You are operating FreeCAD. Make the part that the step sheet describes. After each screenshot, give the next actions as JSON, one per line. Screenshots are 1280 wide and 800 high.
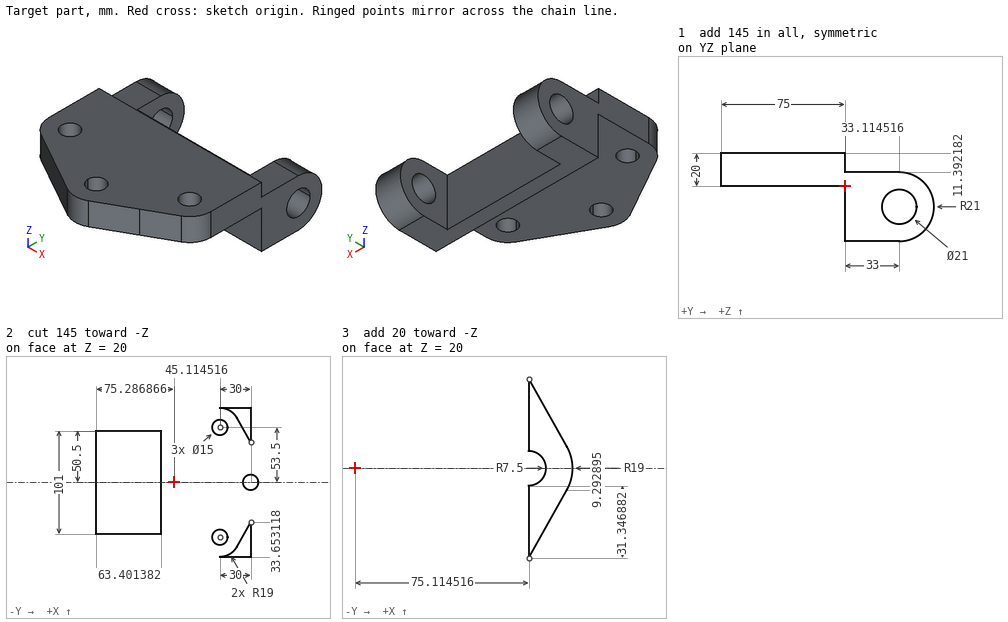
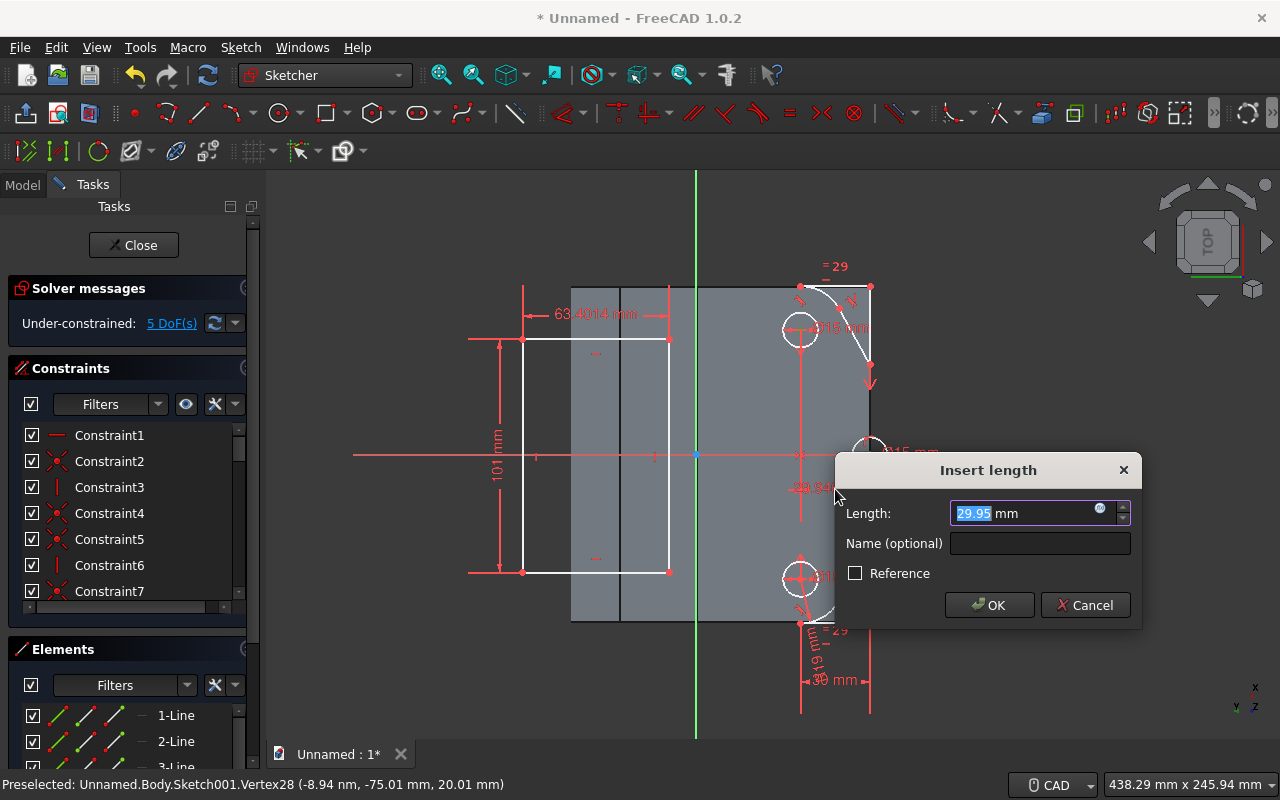
{"action": "type", "text": "30"}
{"action": "key", "text": "Return"}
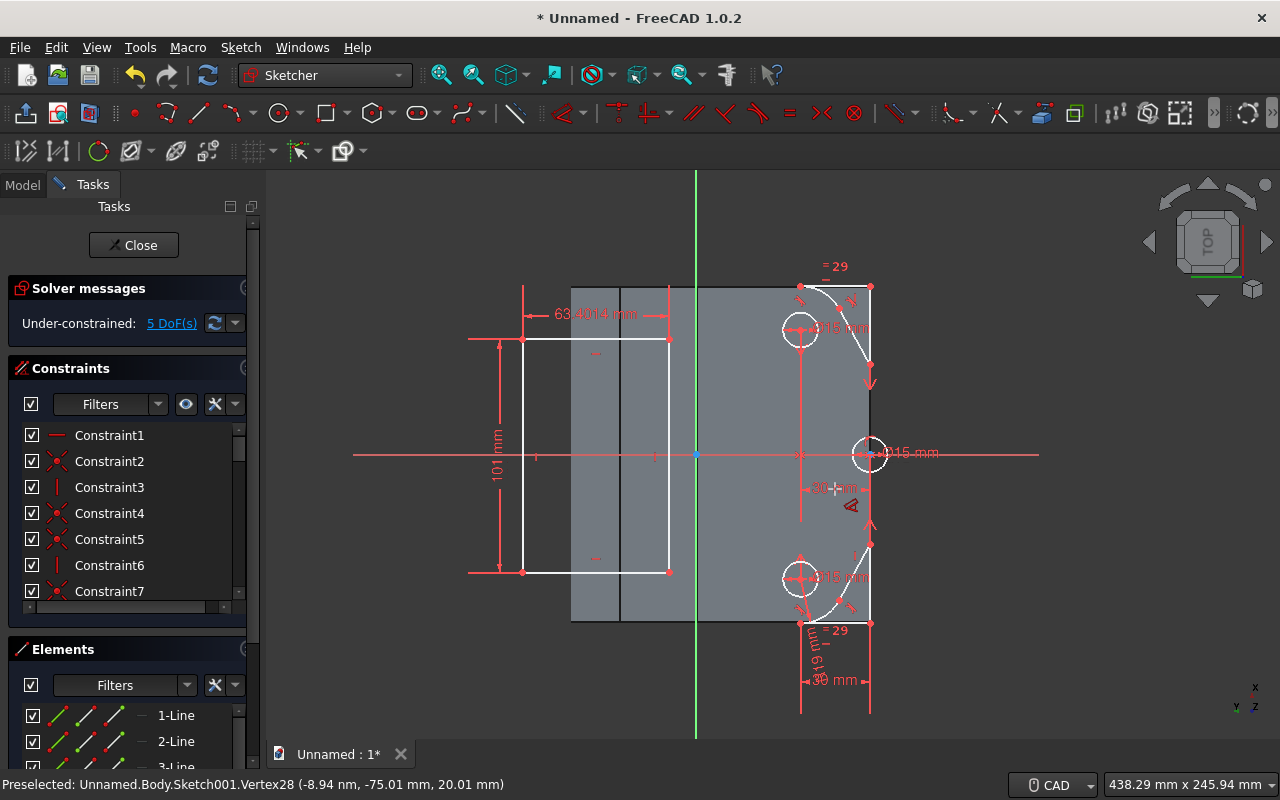
{"action": "left_click", "coordinate": [801, 330]}
{"action": "left_click", "coordinate": [835, 392]}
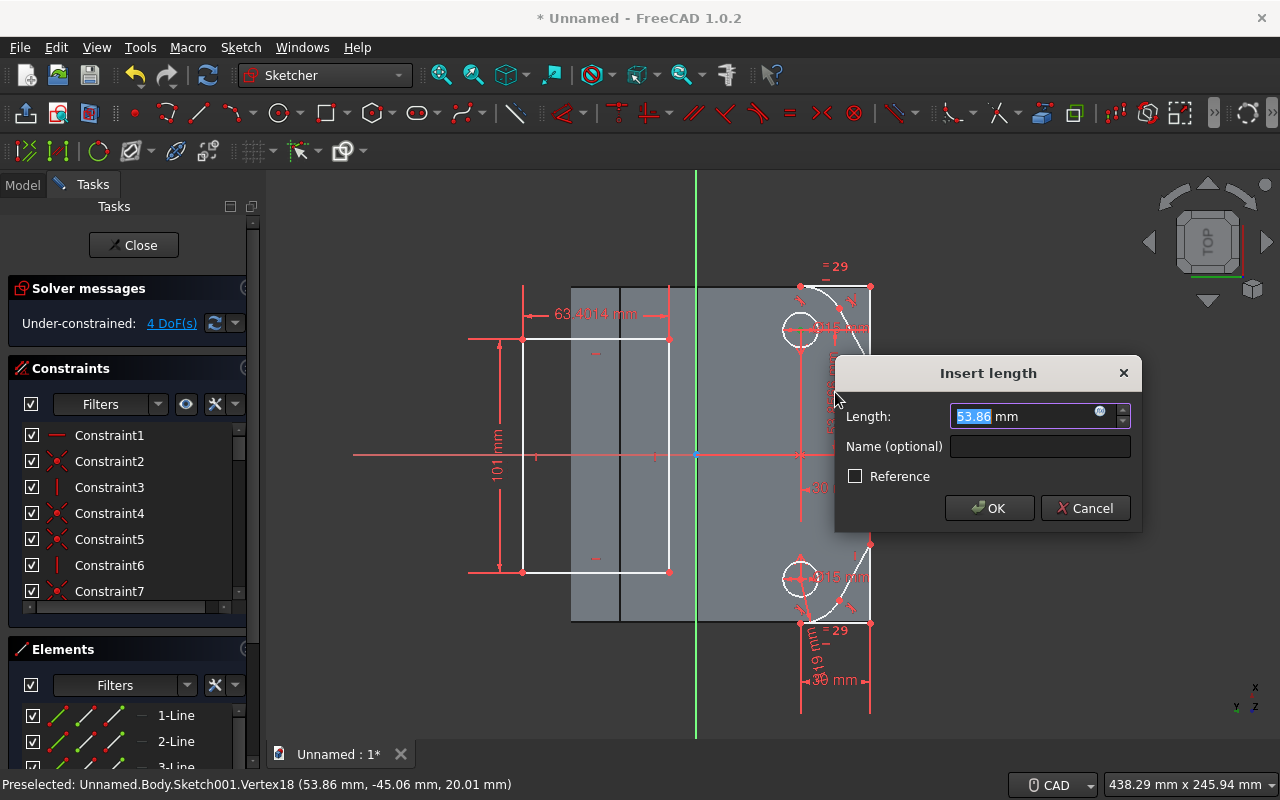
{"action": "type", "text": "53.5"}
{"action": "key", "text": "Return"}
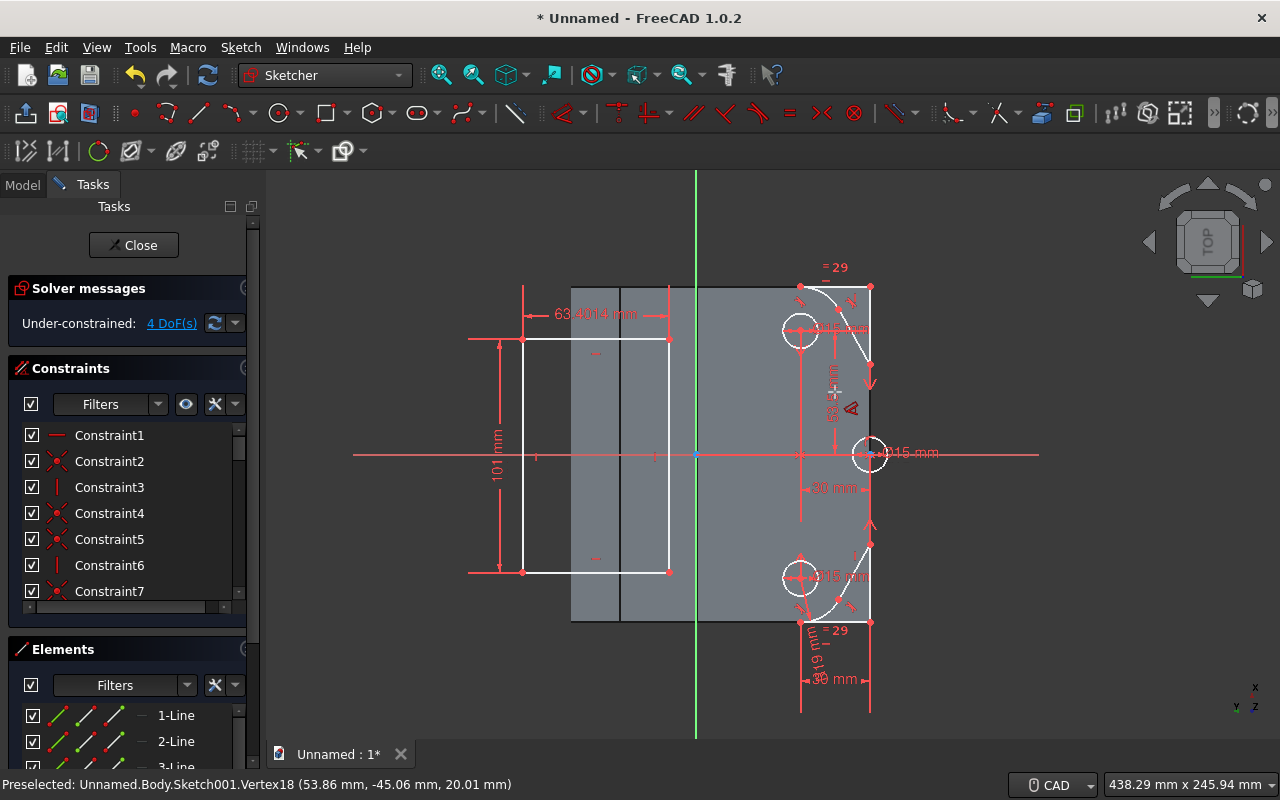
{"action": "left_click", "coordinate": [523, 339]}
{"action": "left_click", "coordinate": [489, 397]}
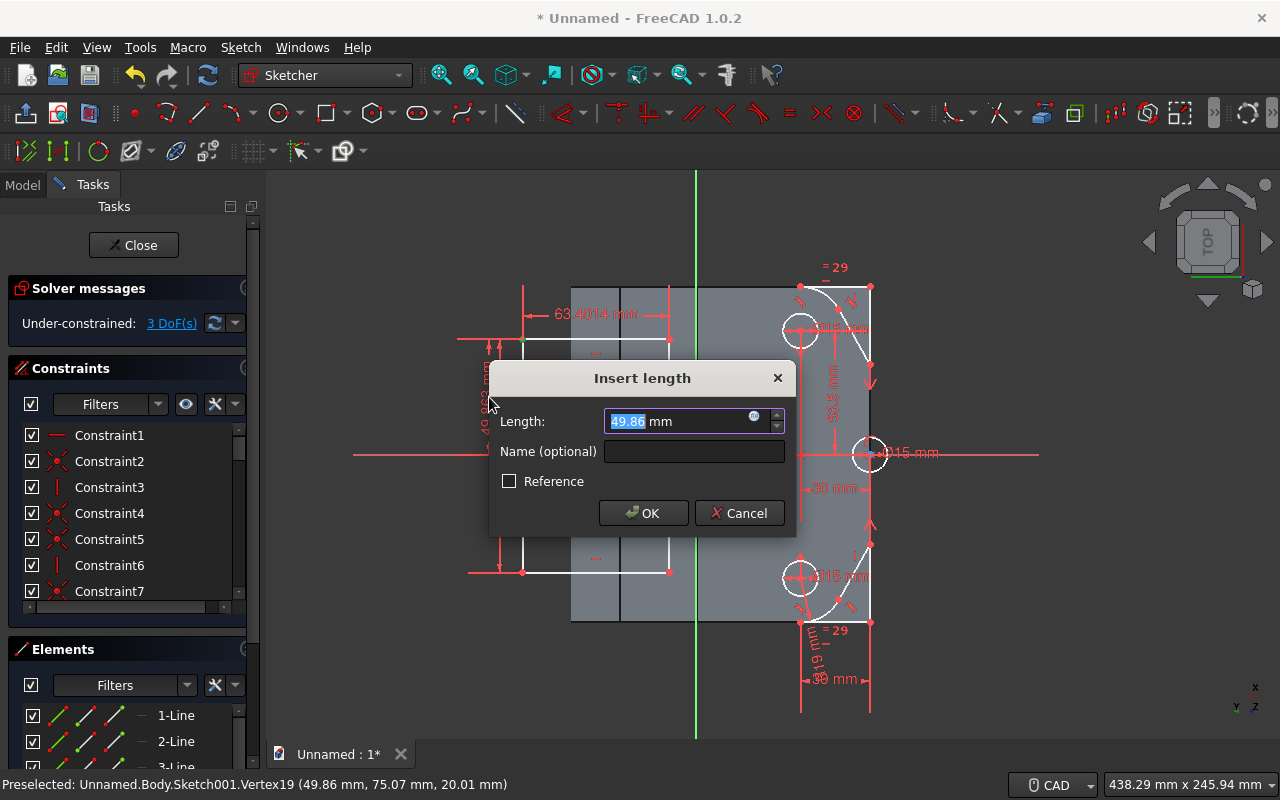
{"action": "type", "text": "50.5"}
{"action": "key", "text": "Return"}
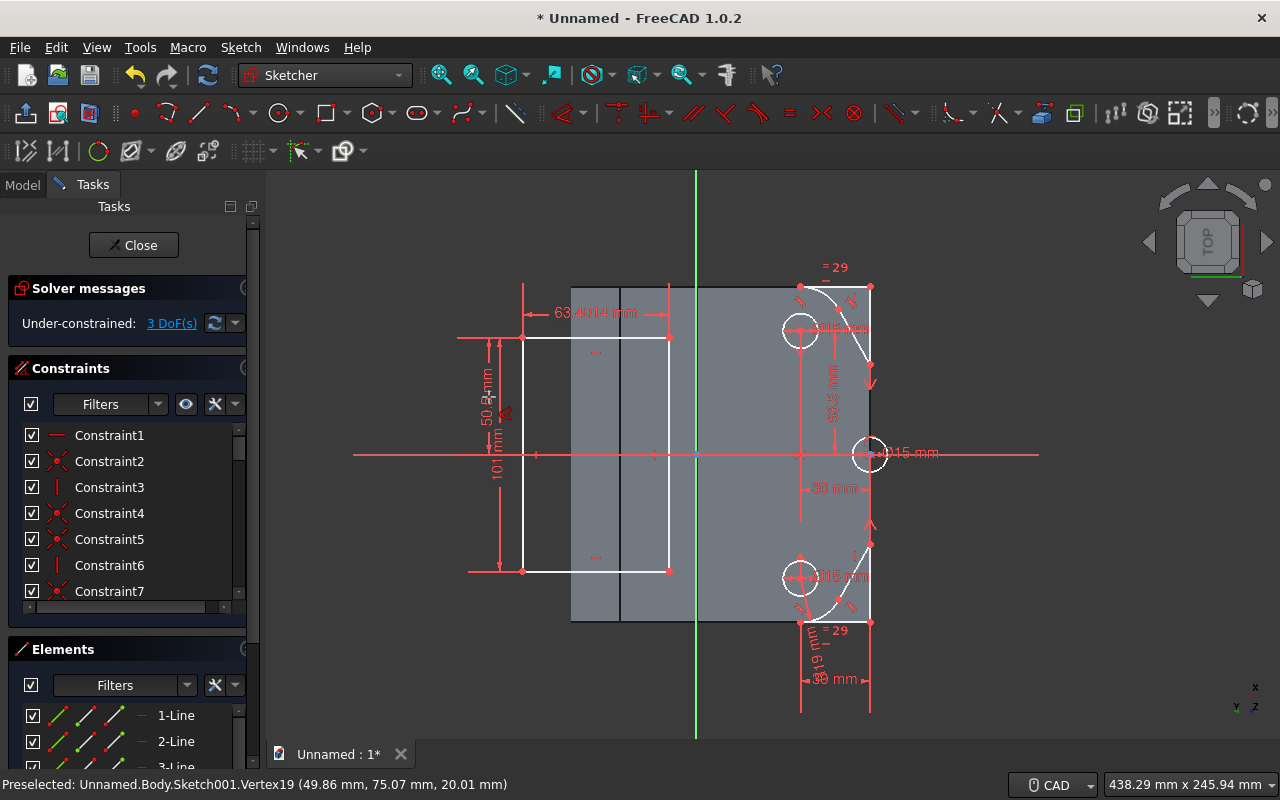
{"action": "left_click", "coordinate": [870, 599]}
{"action": "left_click", "coordinate": [904, 583]}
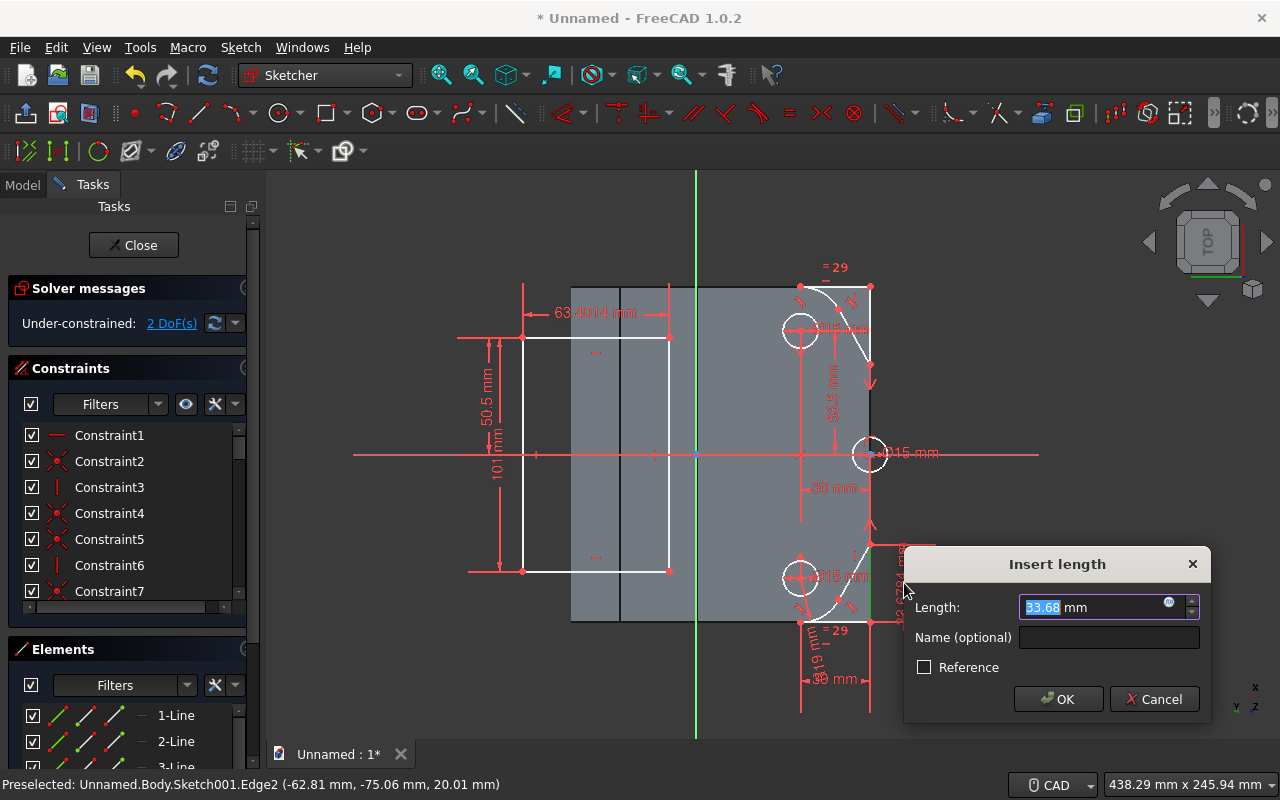
{"action": "type", "text": "33.653118"}
{"action": "key", "text": "Return"}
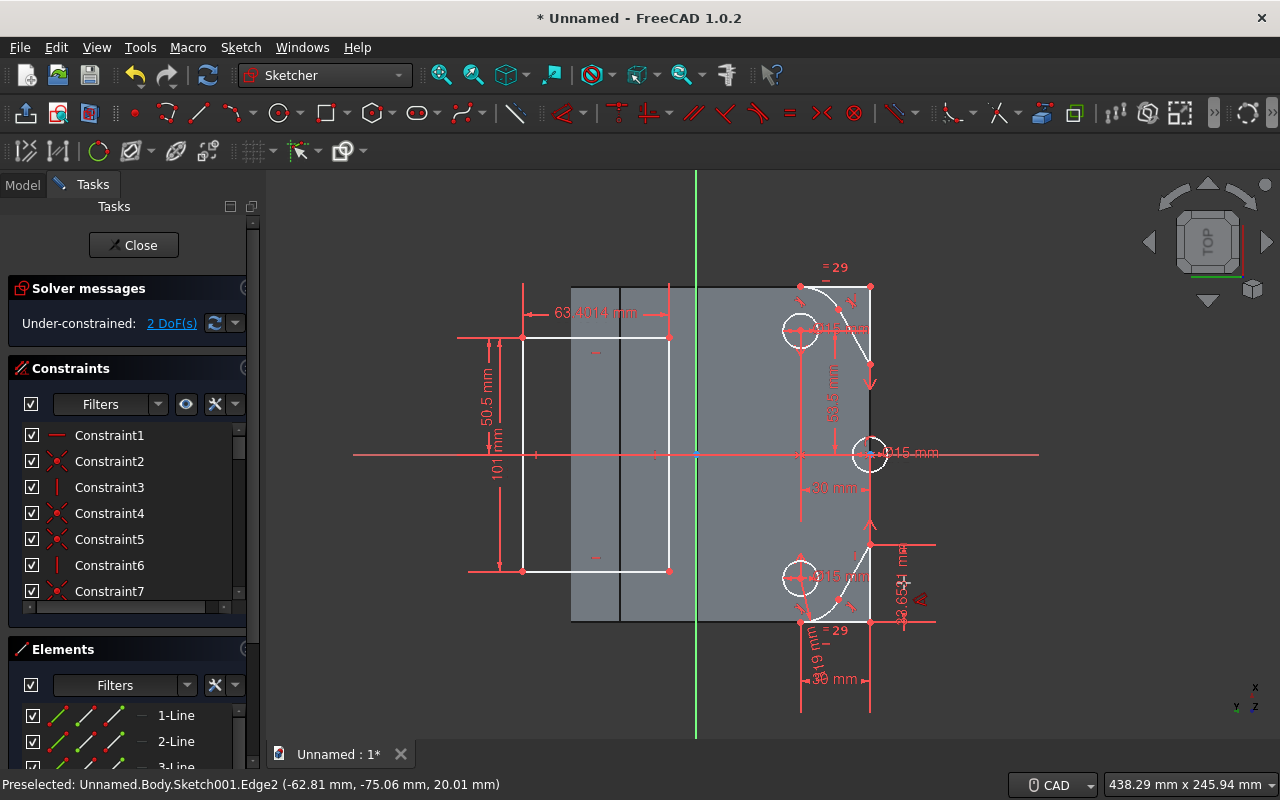
{"action": "left_click", "coordinate": [801, 331]}
{"action": "left_click", "coordinate": [748, 297]}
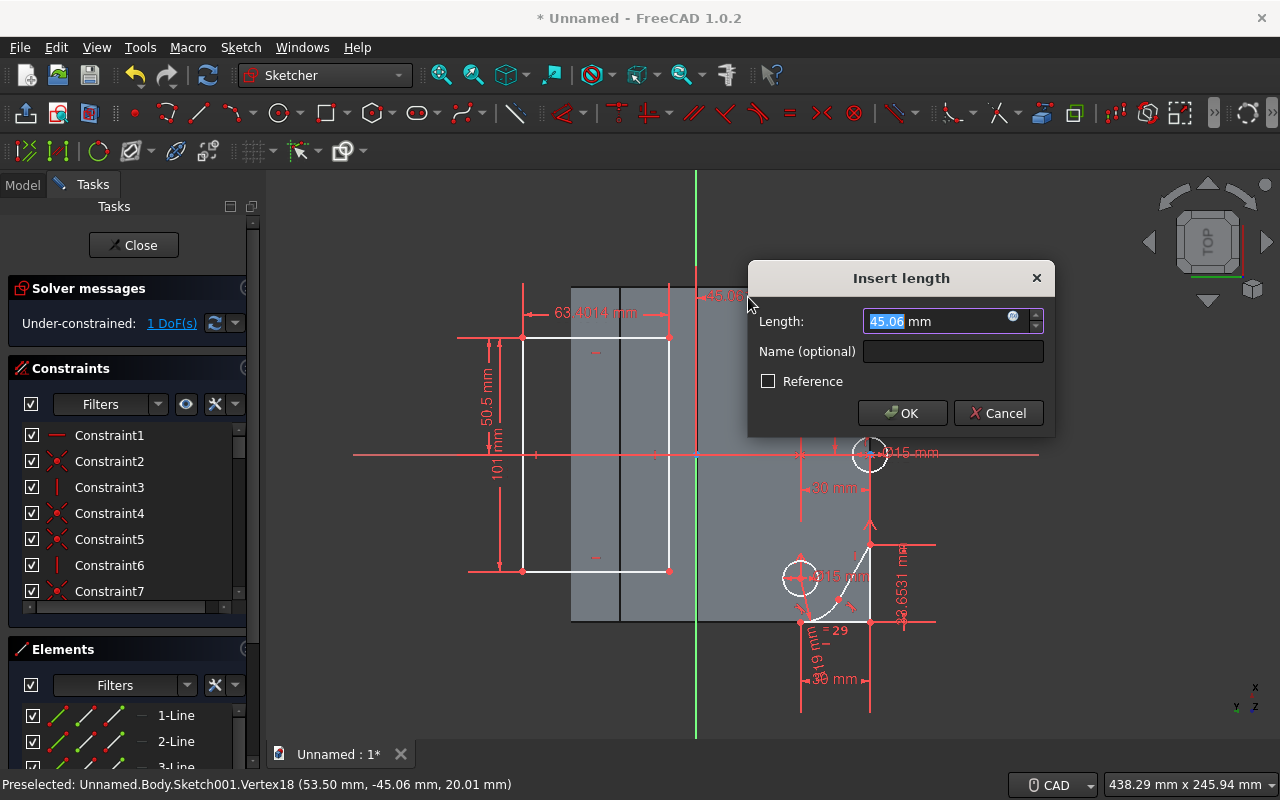
{"action": "type", "text": "45.114516"}
{"action": "key", "text": "Return"}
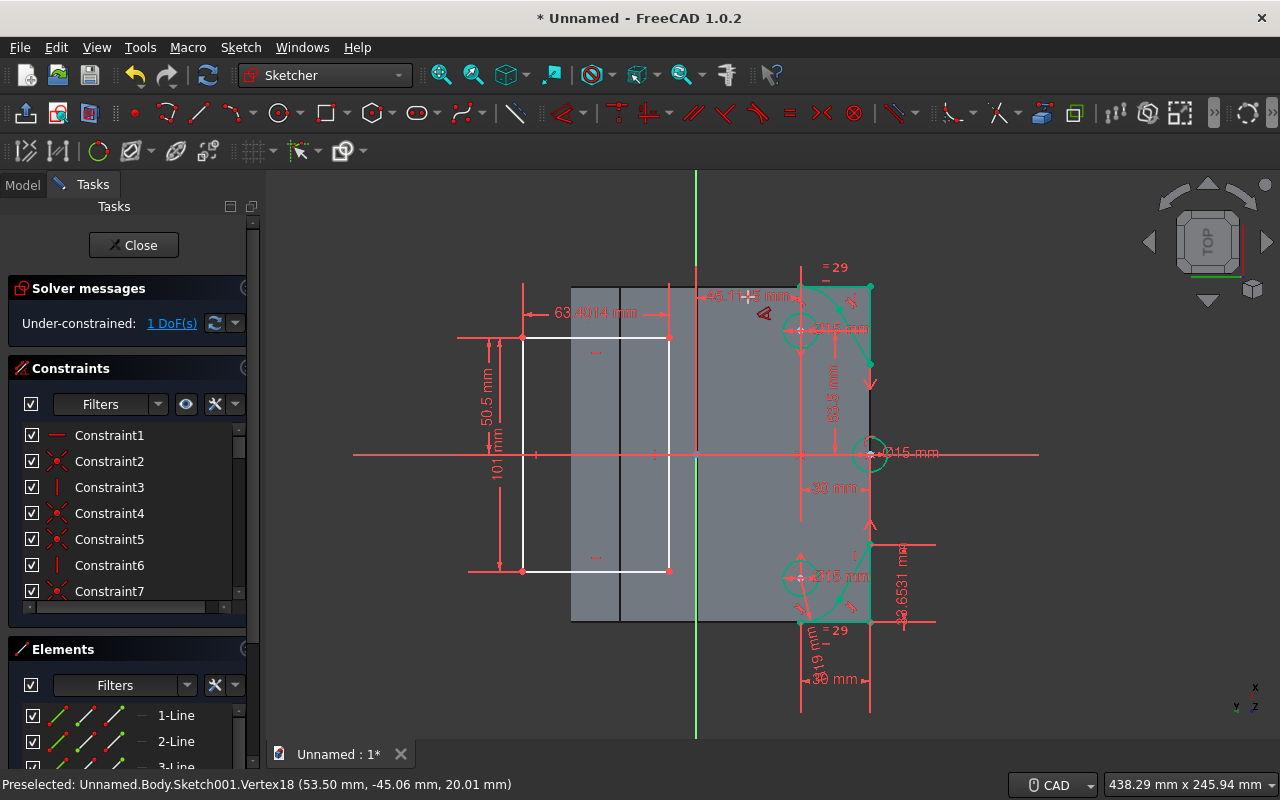
{"action": "left_click", "coordinate": [523, 338]}
{"action": "left_click", "coordinate": [610, 304]}